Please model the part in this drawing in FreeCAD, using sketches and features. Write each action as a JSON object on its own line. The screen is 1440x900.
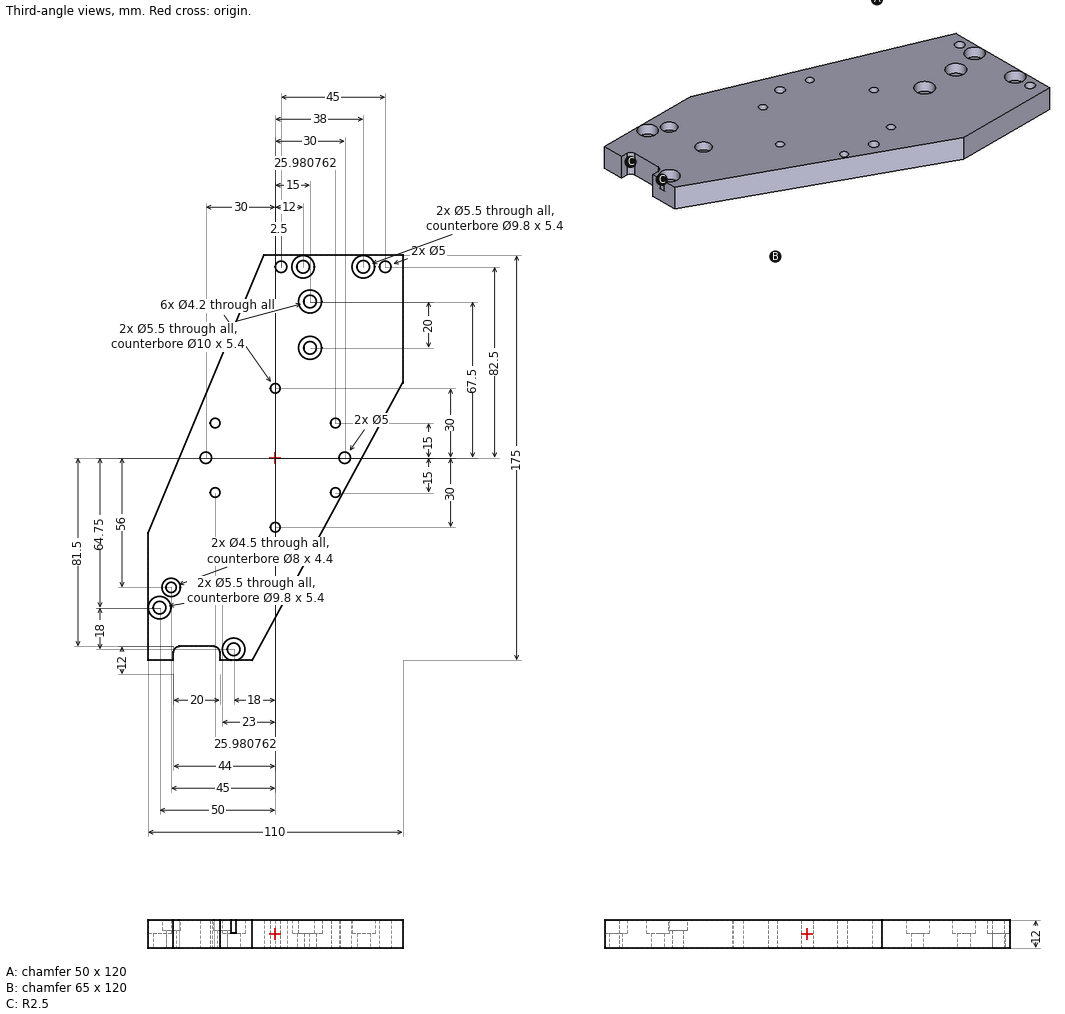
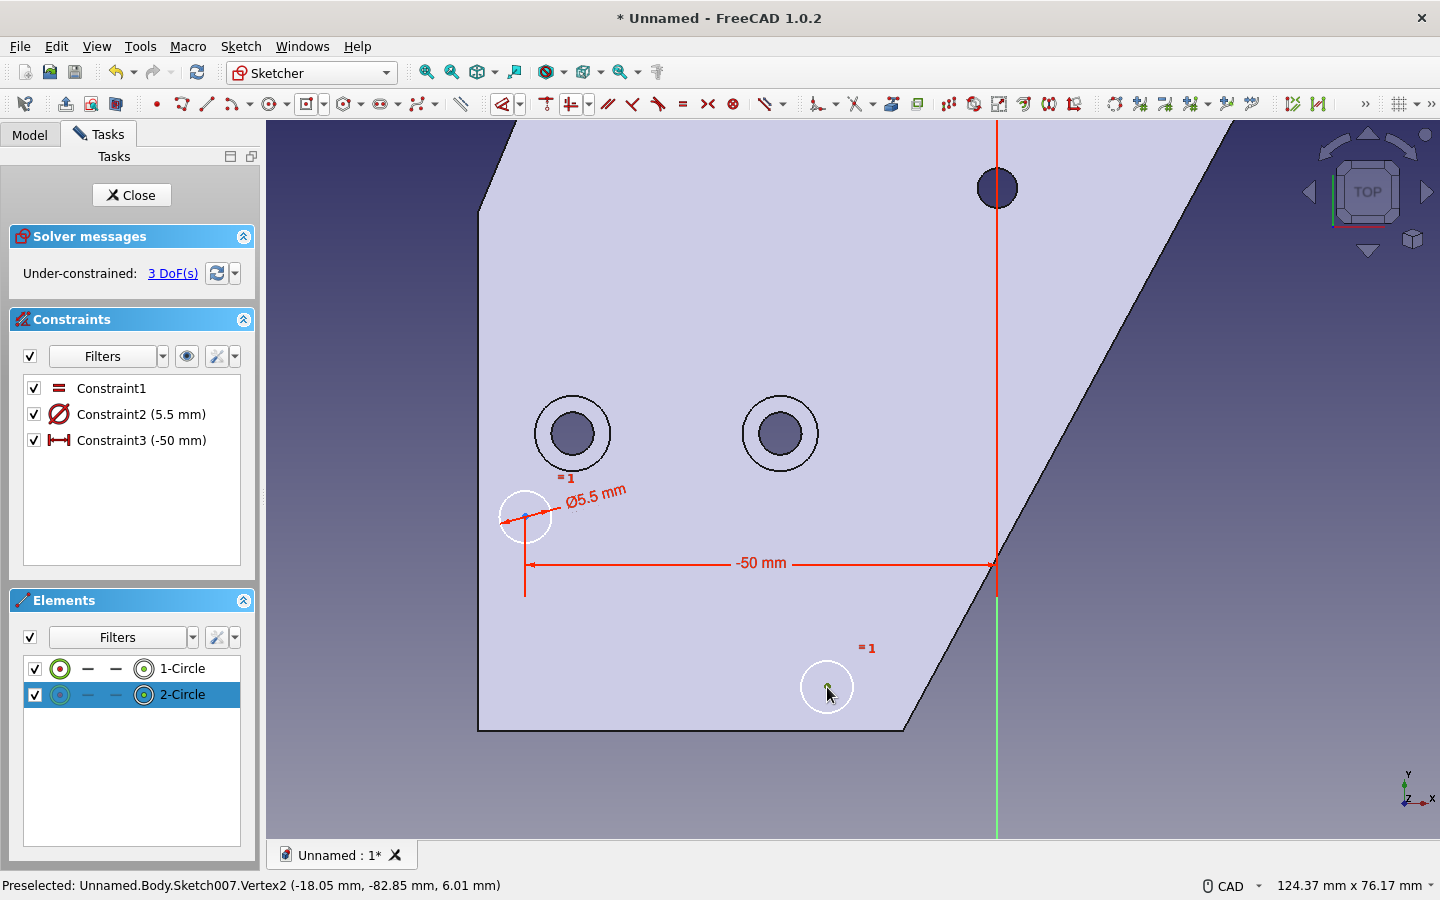
{"action": "left_click", "coordinate": [520, 104]}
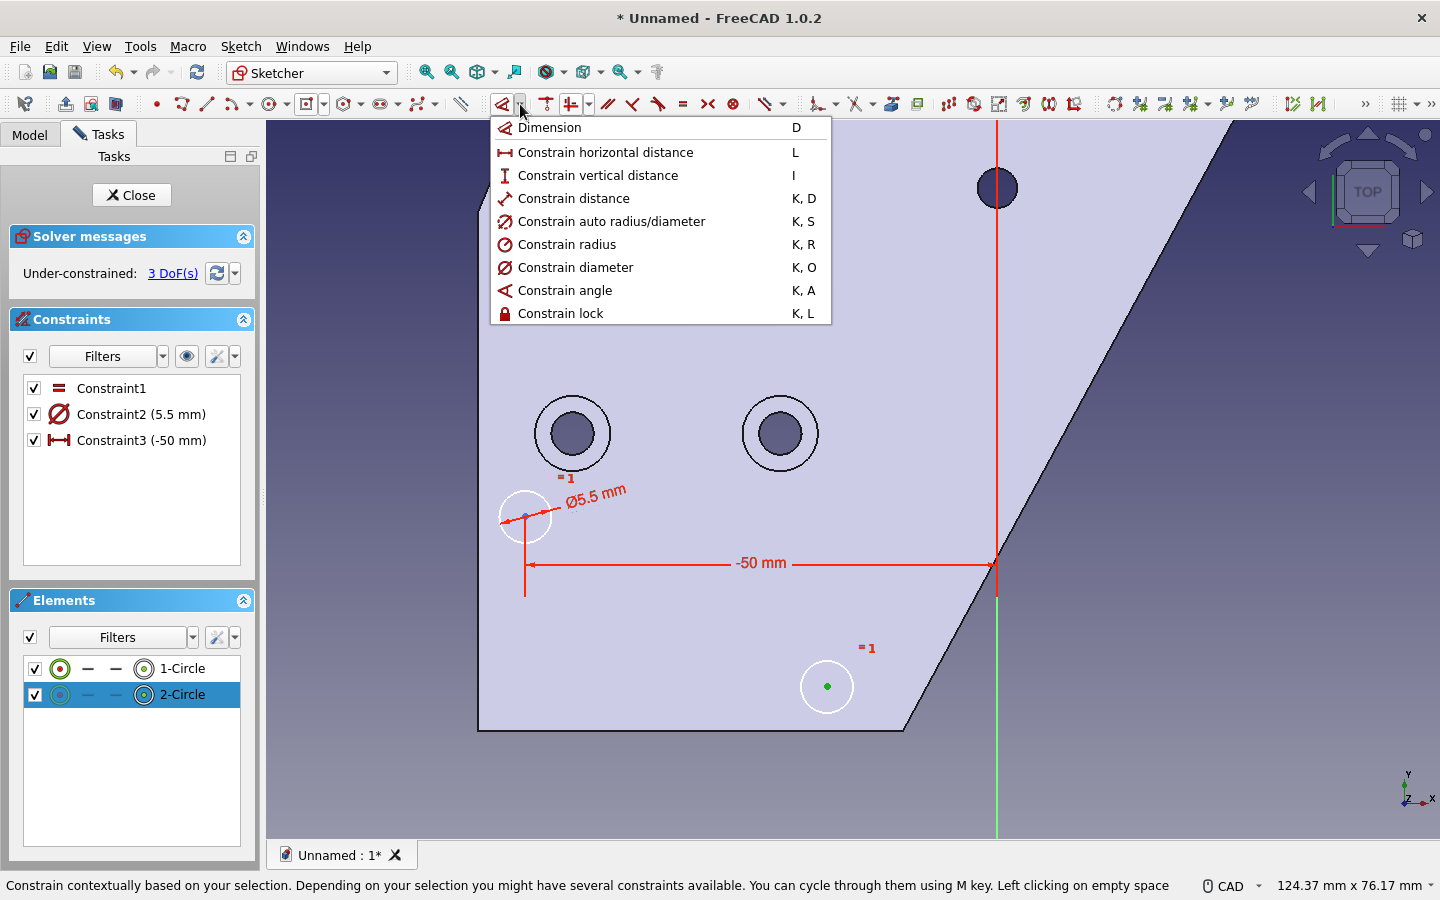
{"action": "left_click", "coordinate": [661, 152]}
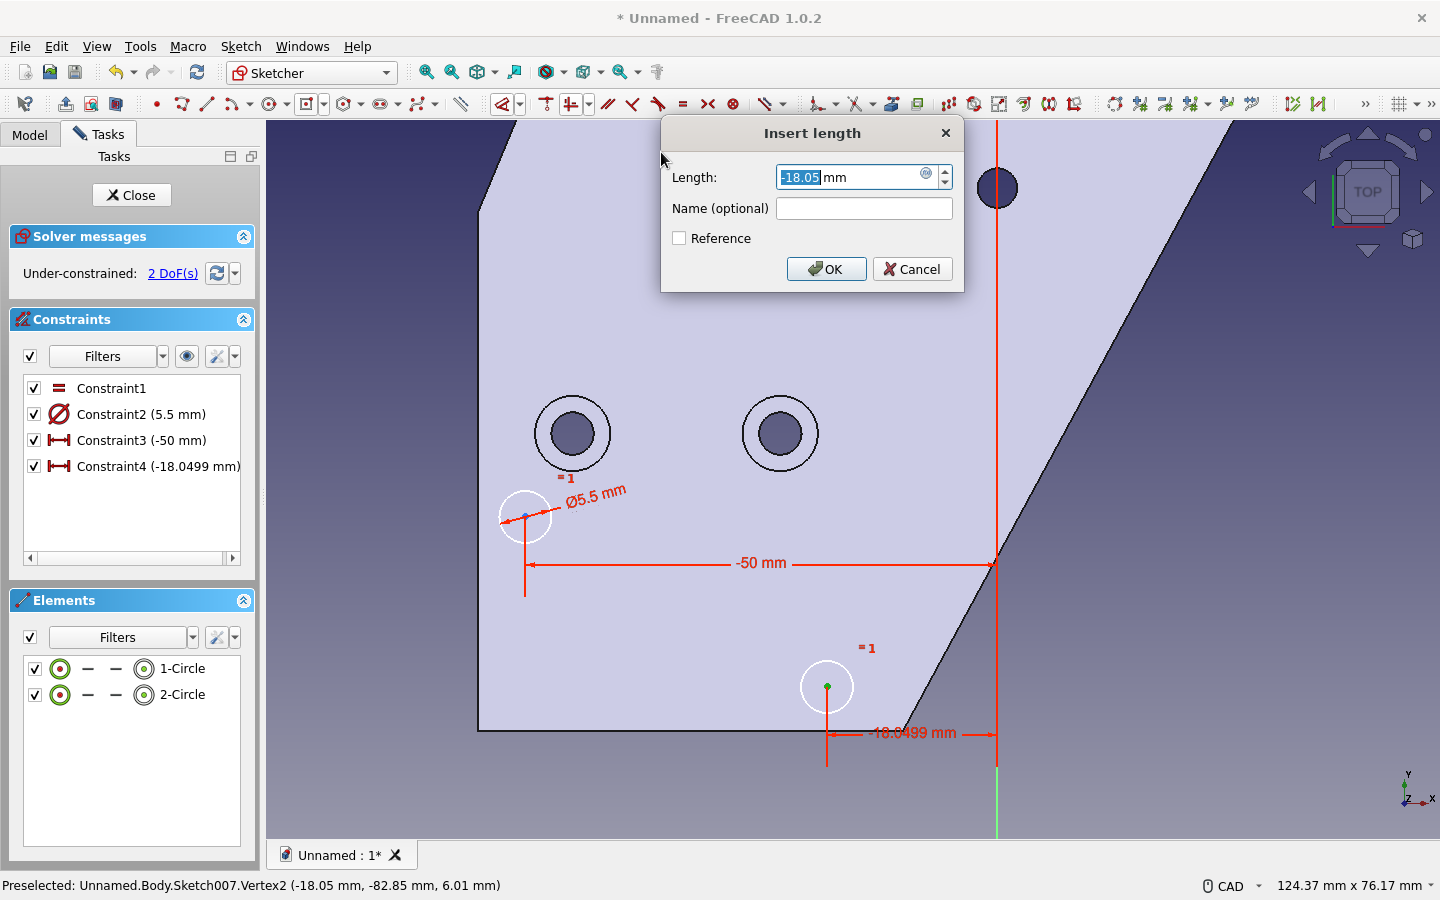
{"action": "type", "text": "-18"}
{"action": "key", "text": "Return"}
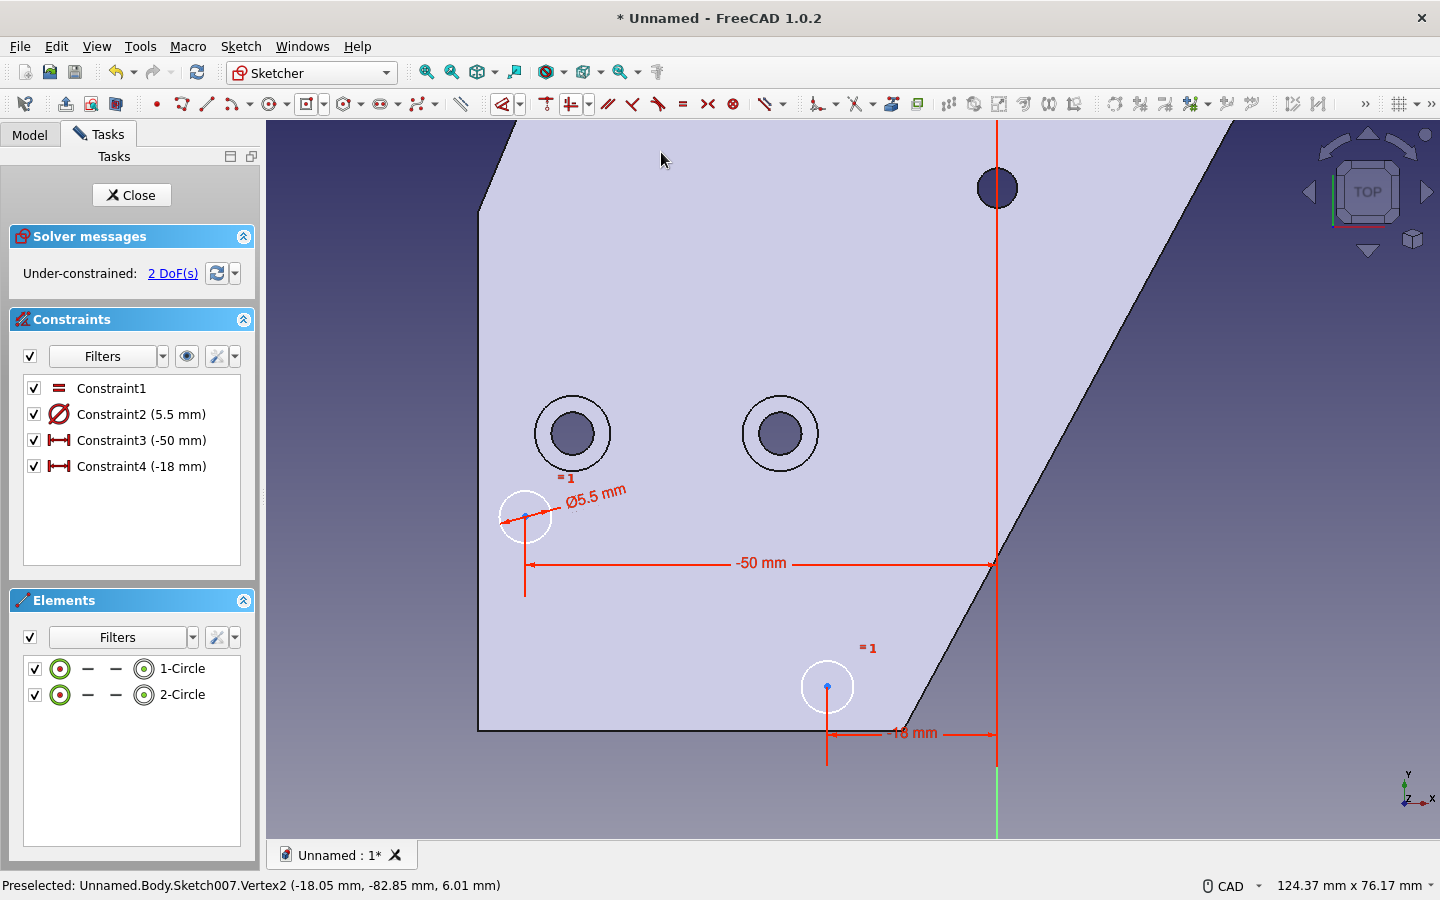
{"action": "left_click", "coordinate": [525, 517]}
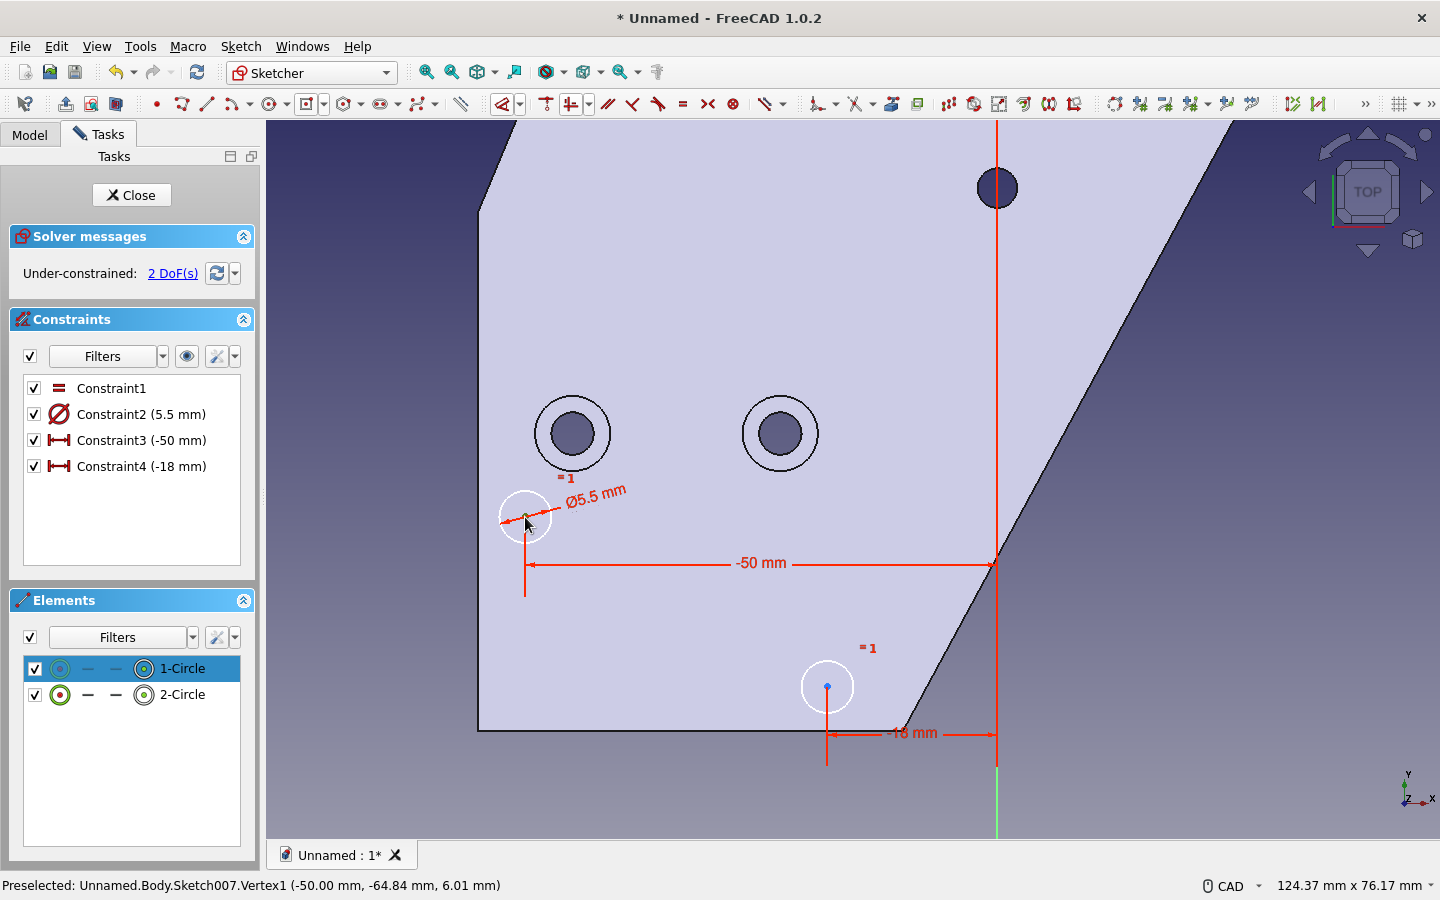
{"action": "left_click", "coordinate": [827, 687]}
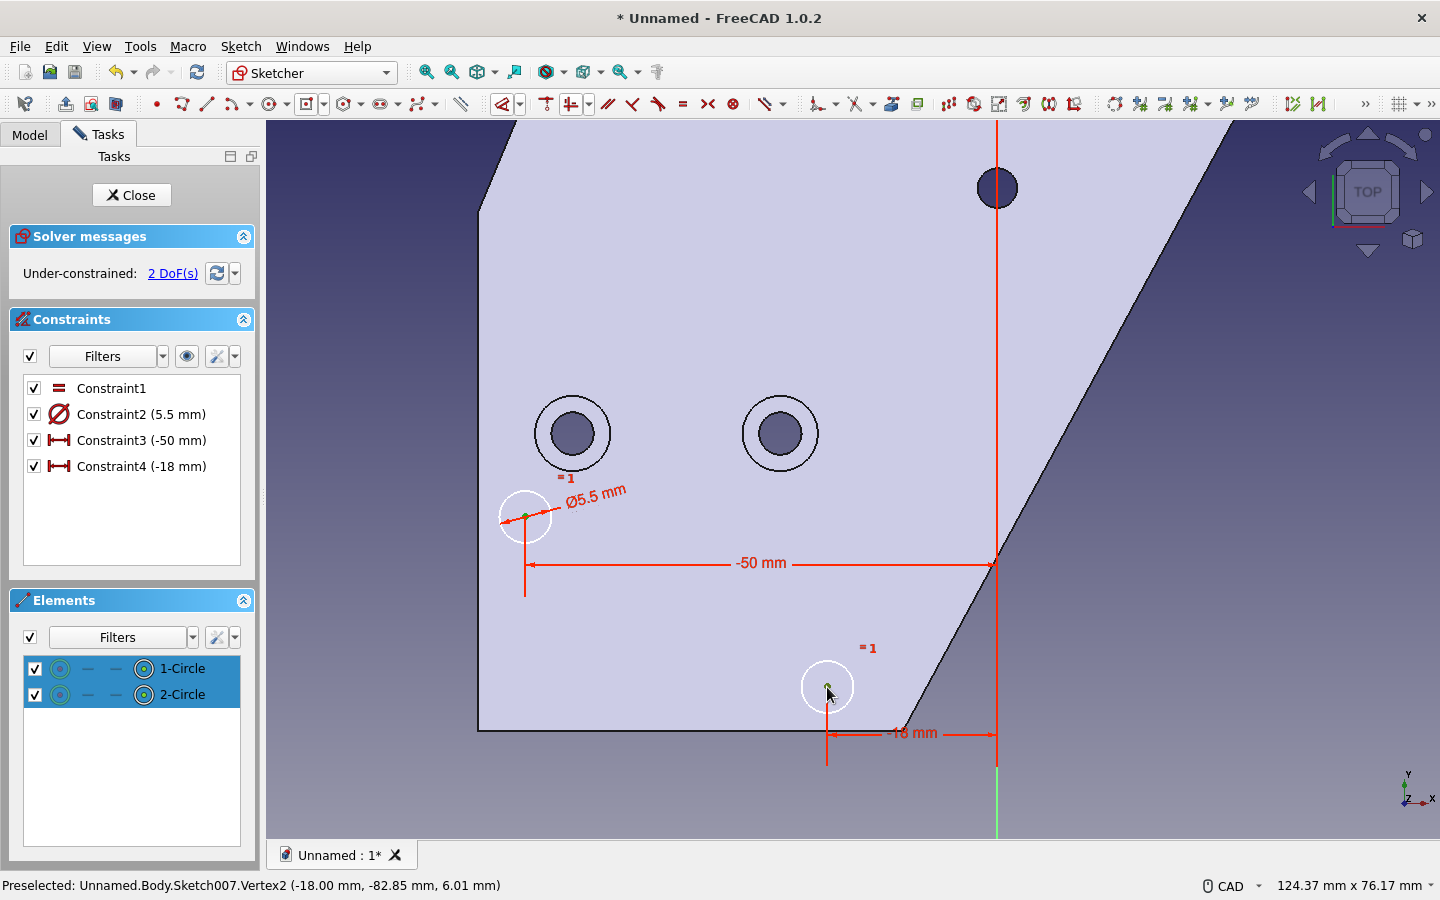
{"action": "key", "text": "i"}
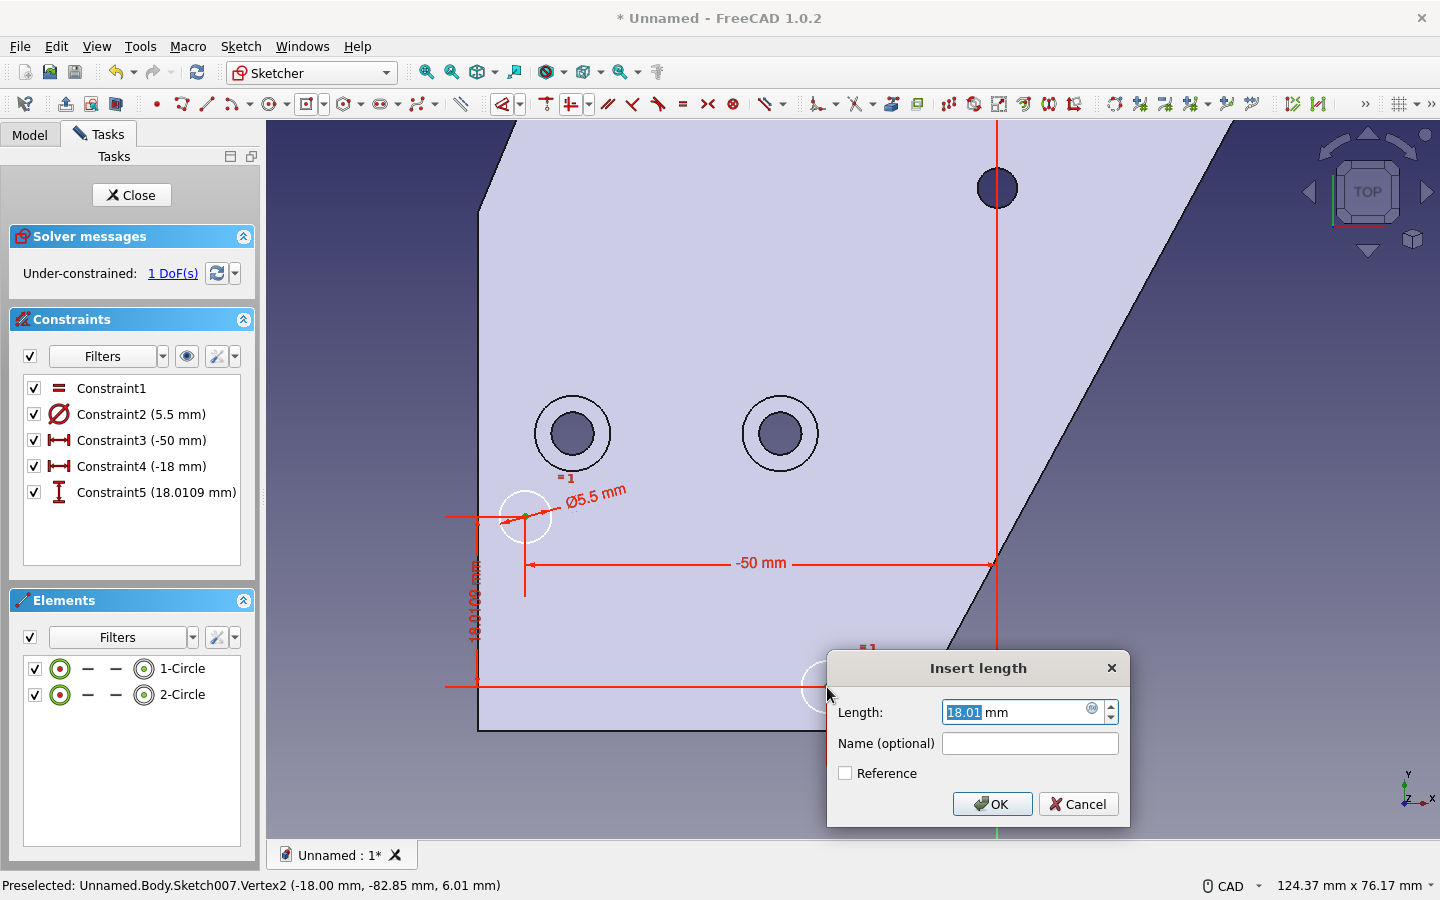
{"action": "type", "text": "18"}
{"action": "key", "text": "Return"}